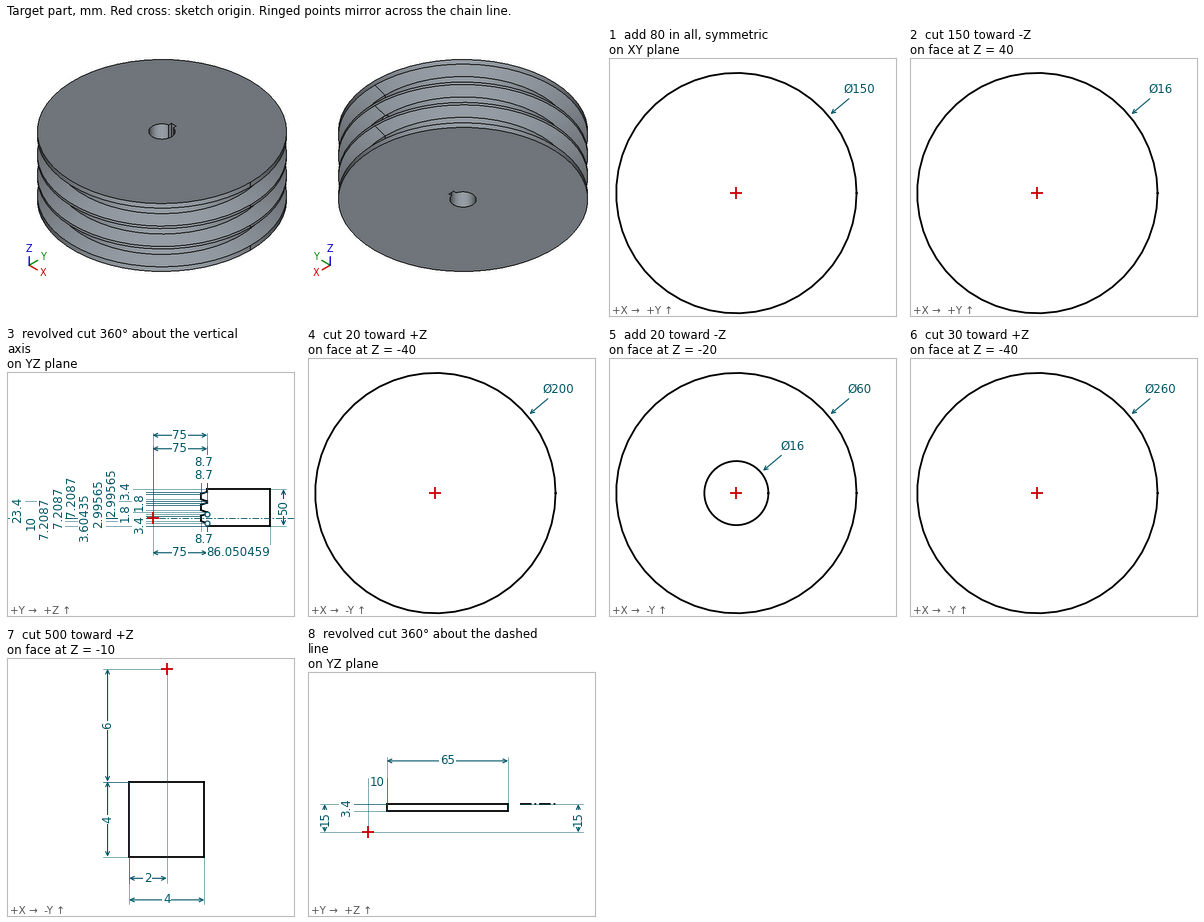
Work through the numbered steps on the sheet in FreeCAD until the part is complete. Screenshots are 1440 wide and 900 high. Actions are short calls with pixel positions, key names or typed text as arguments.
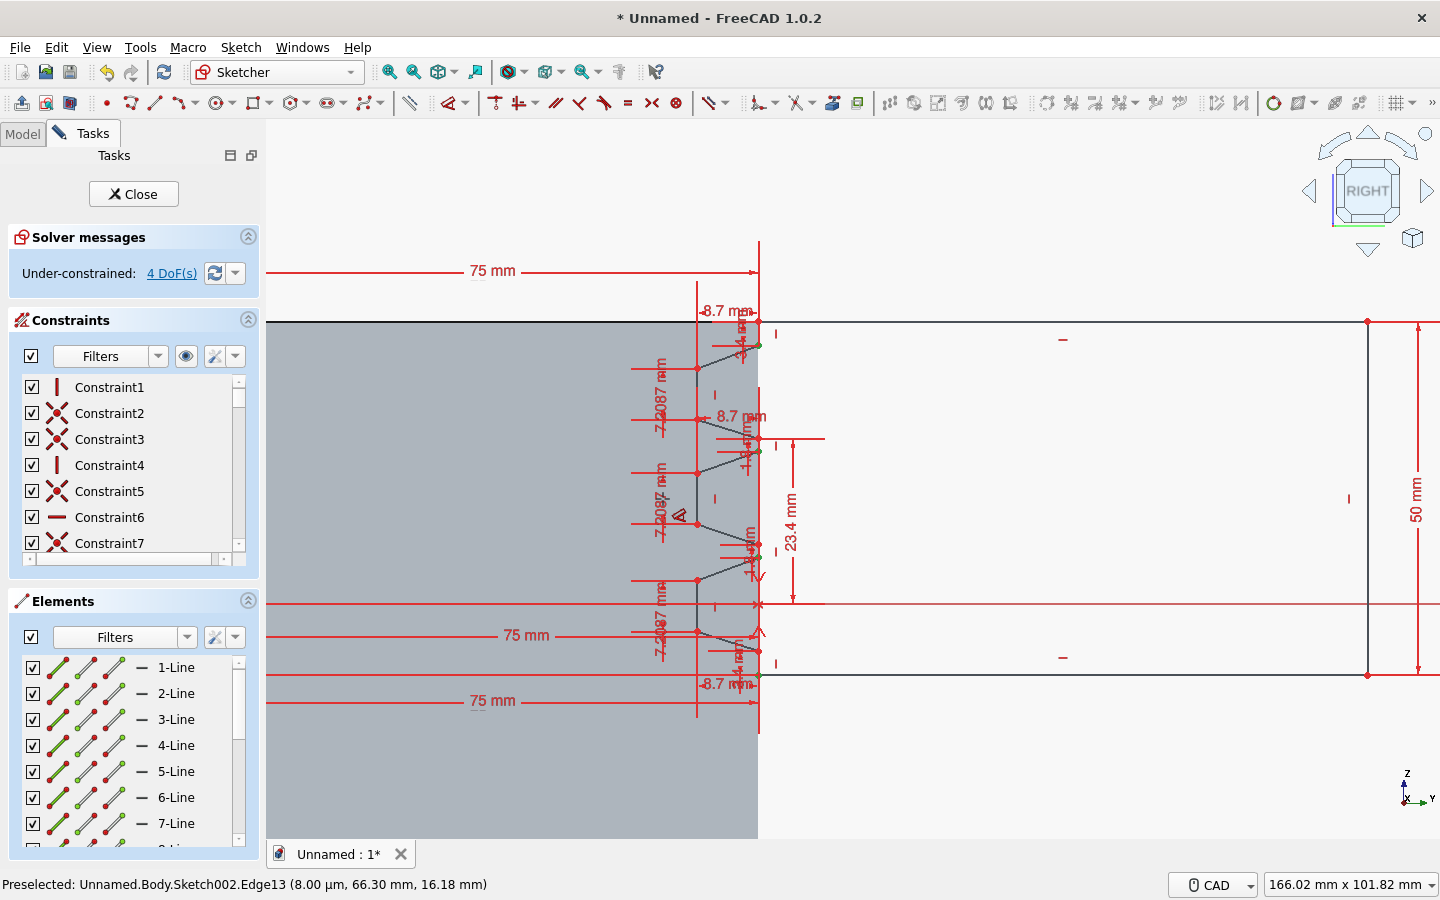
scroll(697, 581, up, 3)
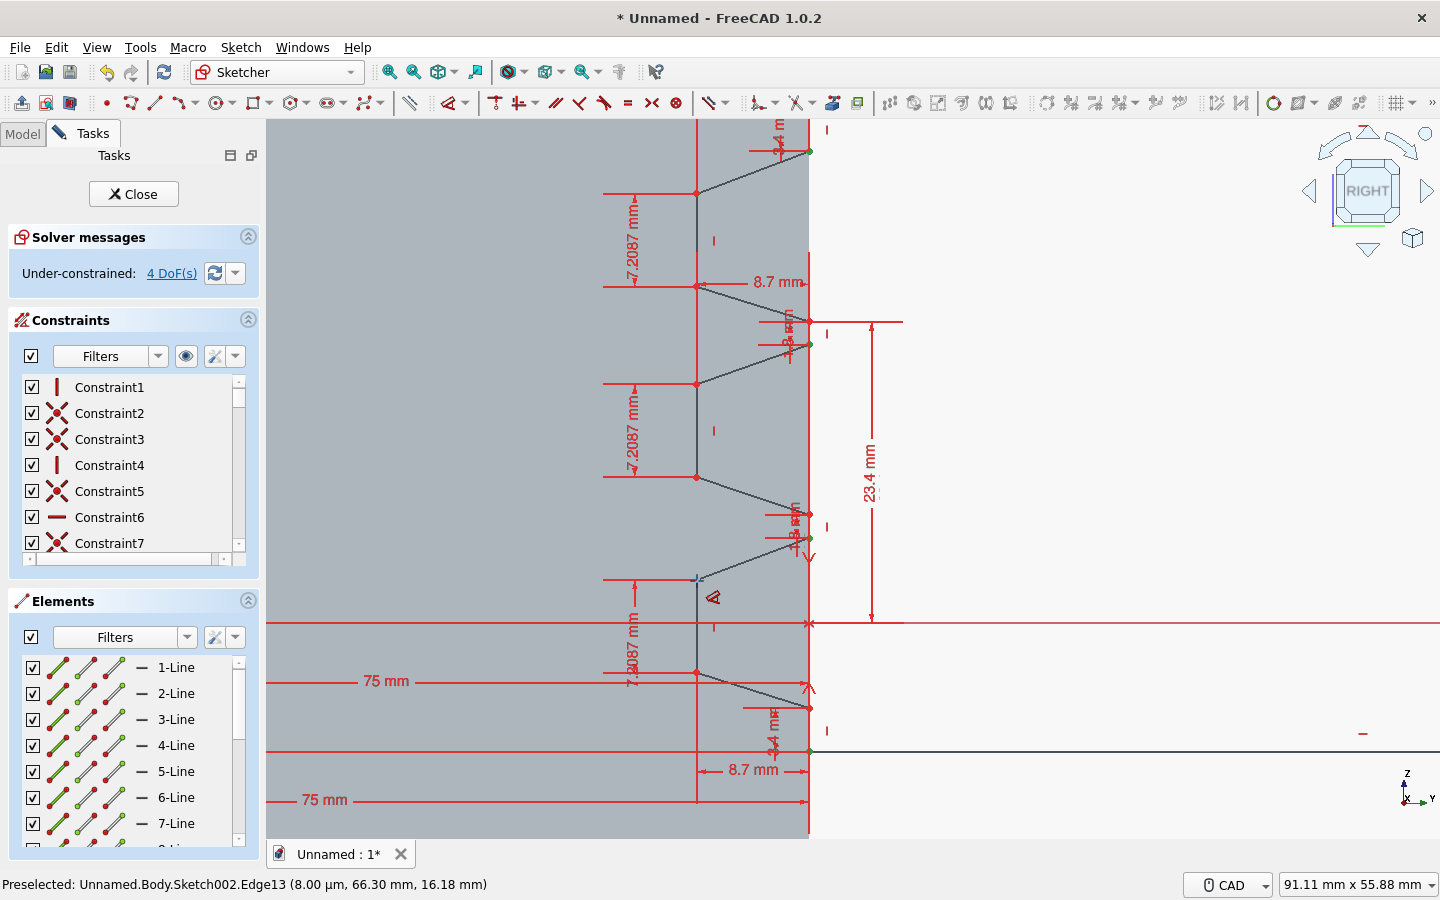
click(697, 580)
click(731, 602)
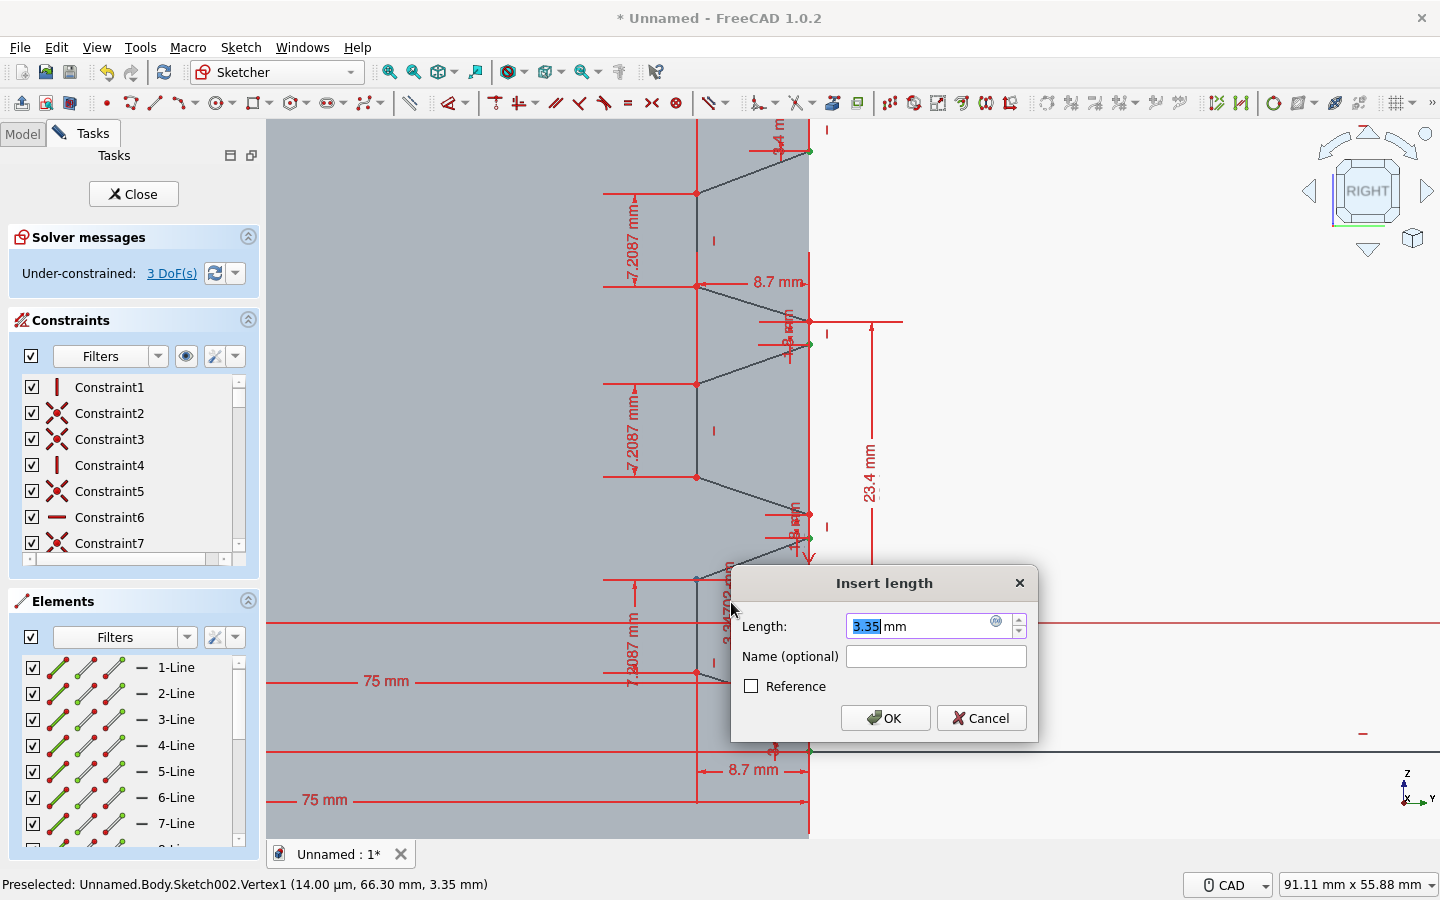
text(3.60435)
key(Return)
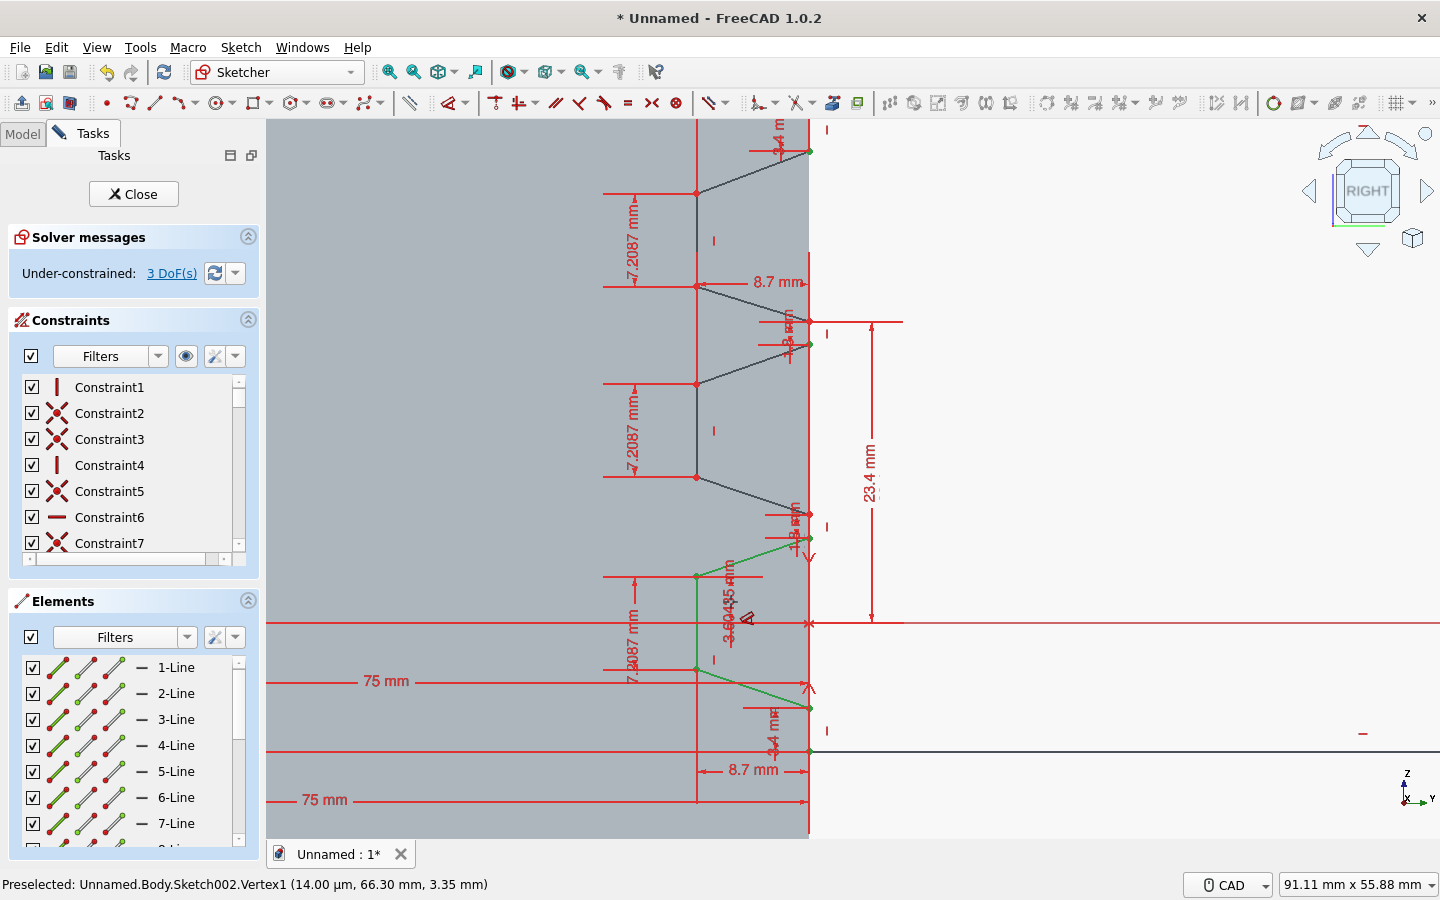
click(775, 164)
click(663, 173)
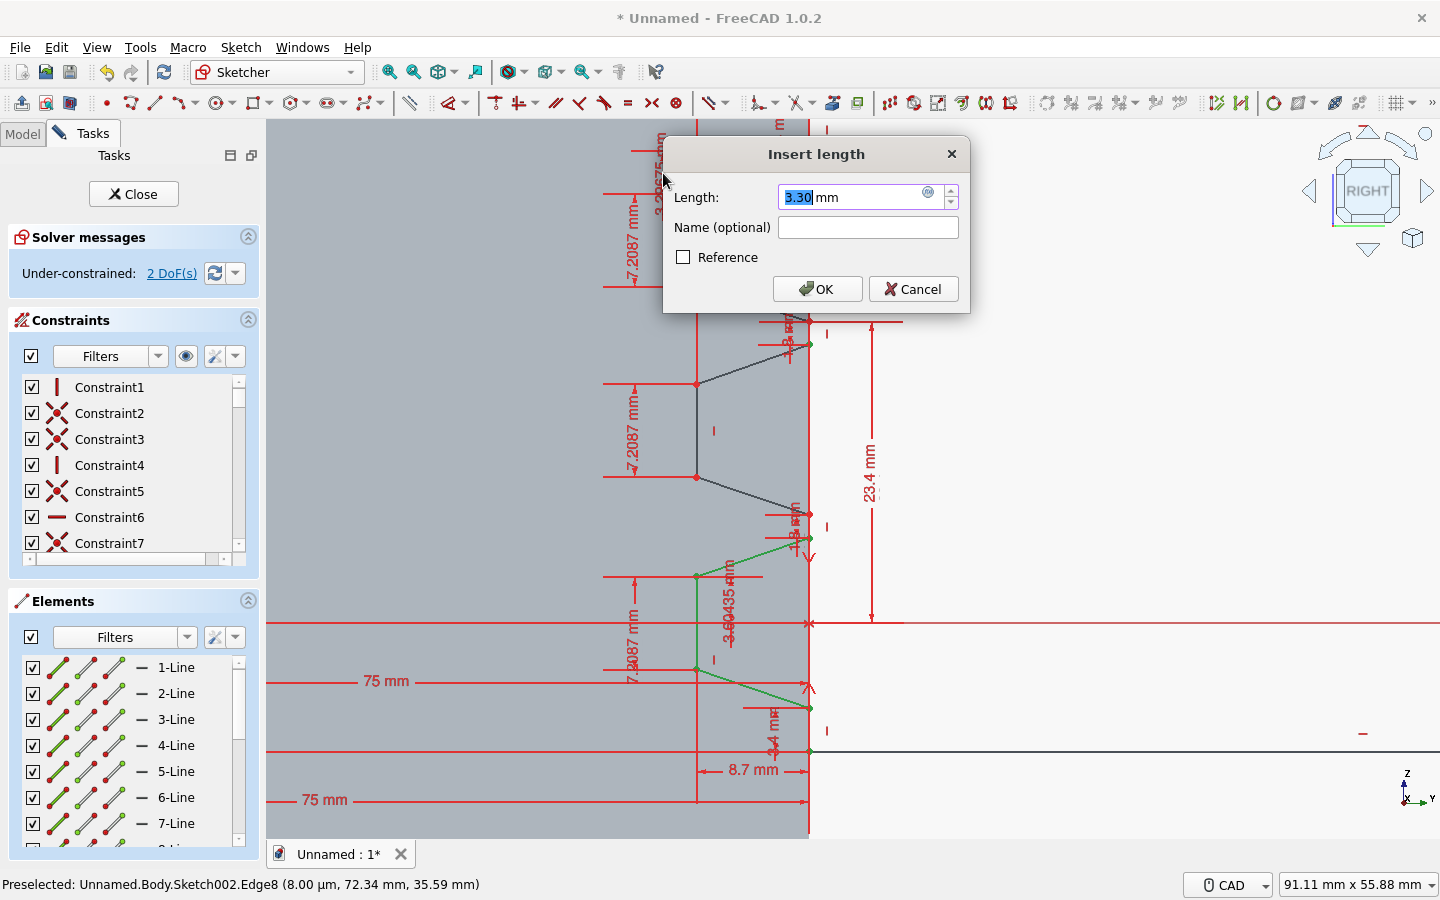
text(2.99565)
key(Return)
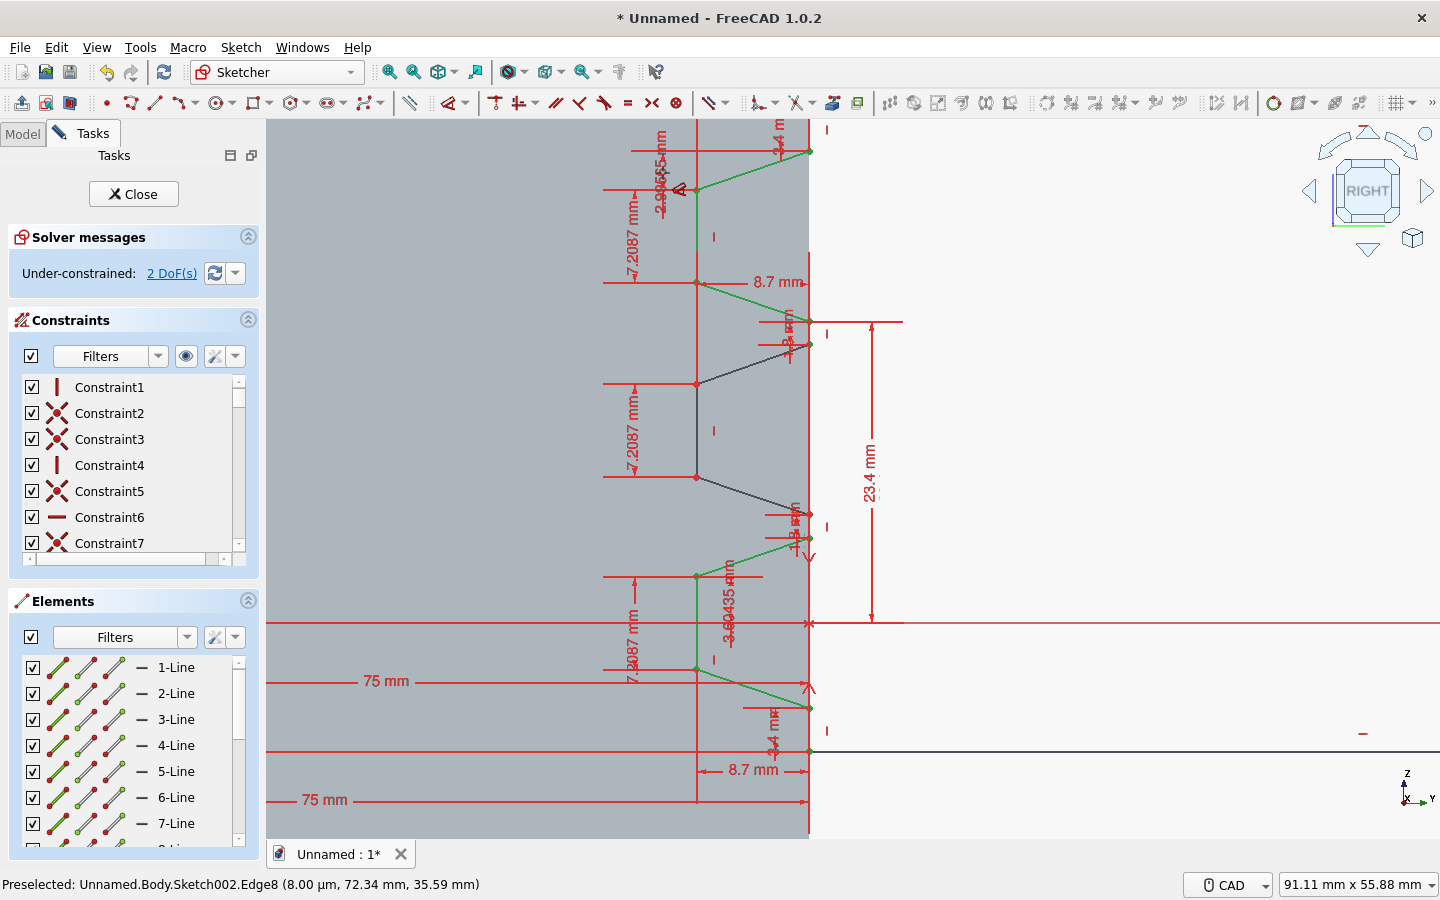
click(775, 357)
click(663, 365)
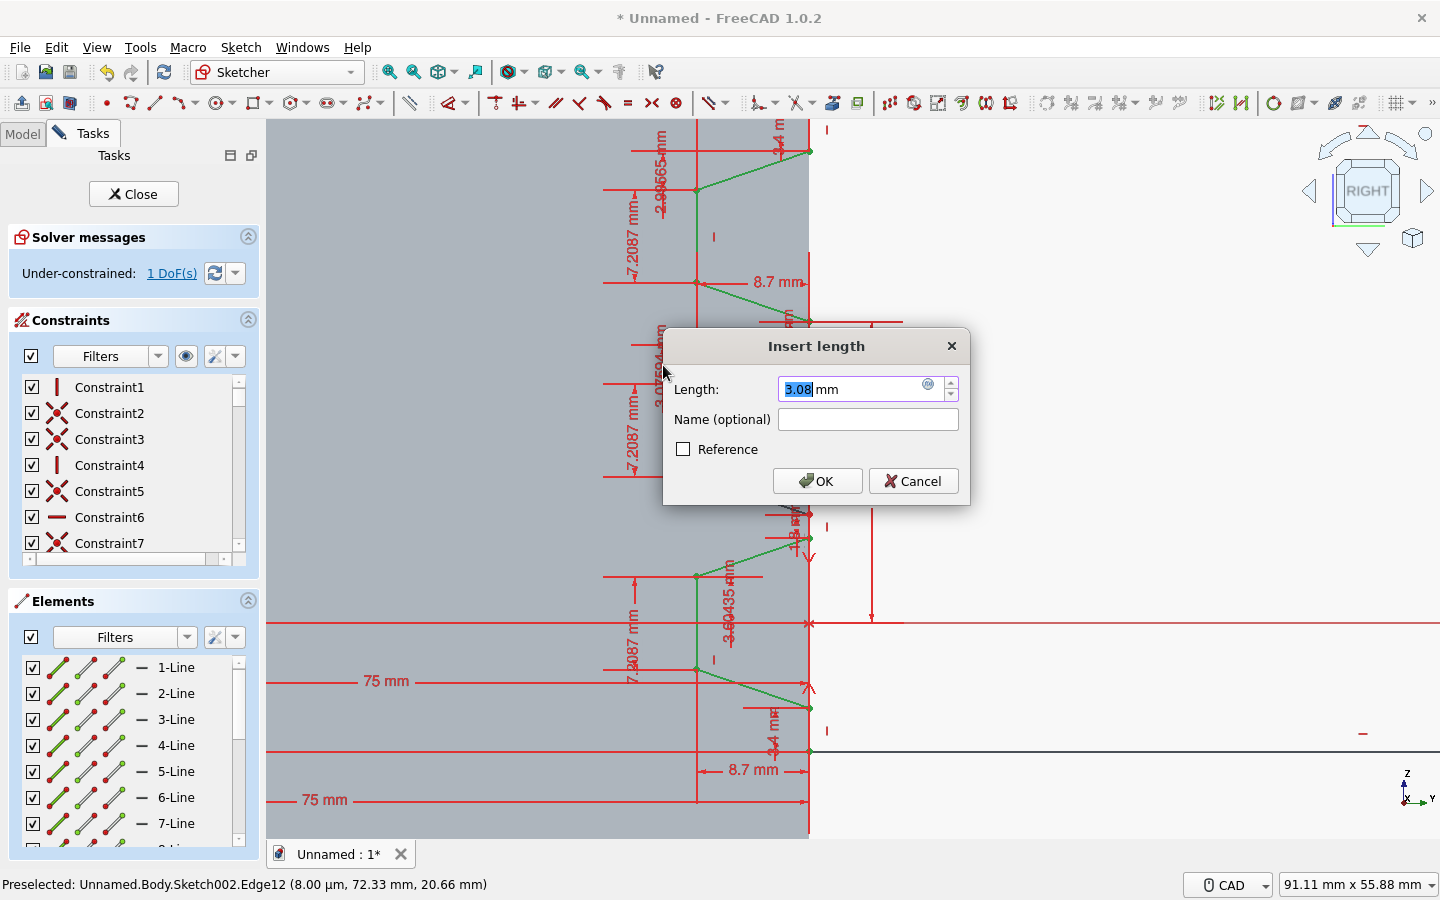
text(2.99565)
key(Return)